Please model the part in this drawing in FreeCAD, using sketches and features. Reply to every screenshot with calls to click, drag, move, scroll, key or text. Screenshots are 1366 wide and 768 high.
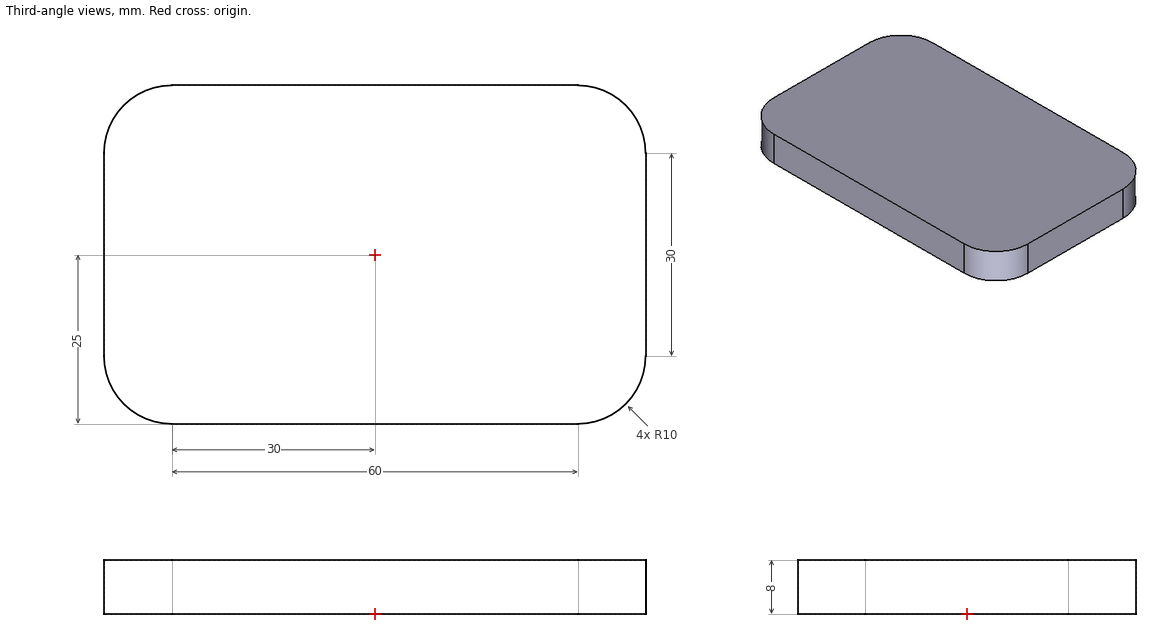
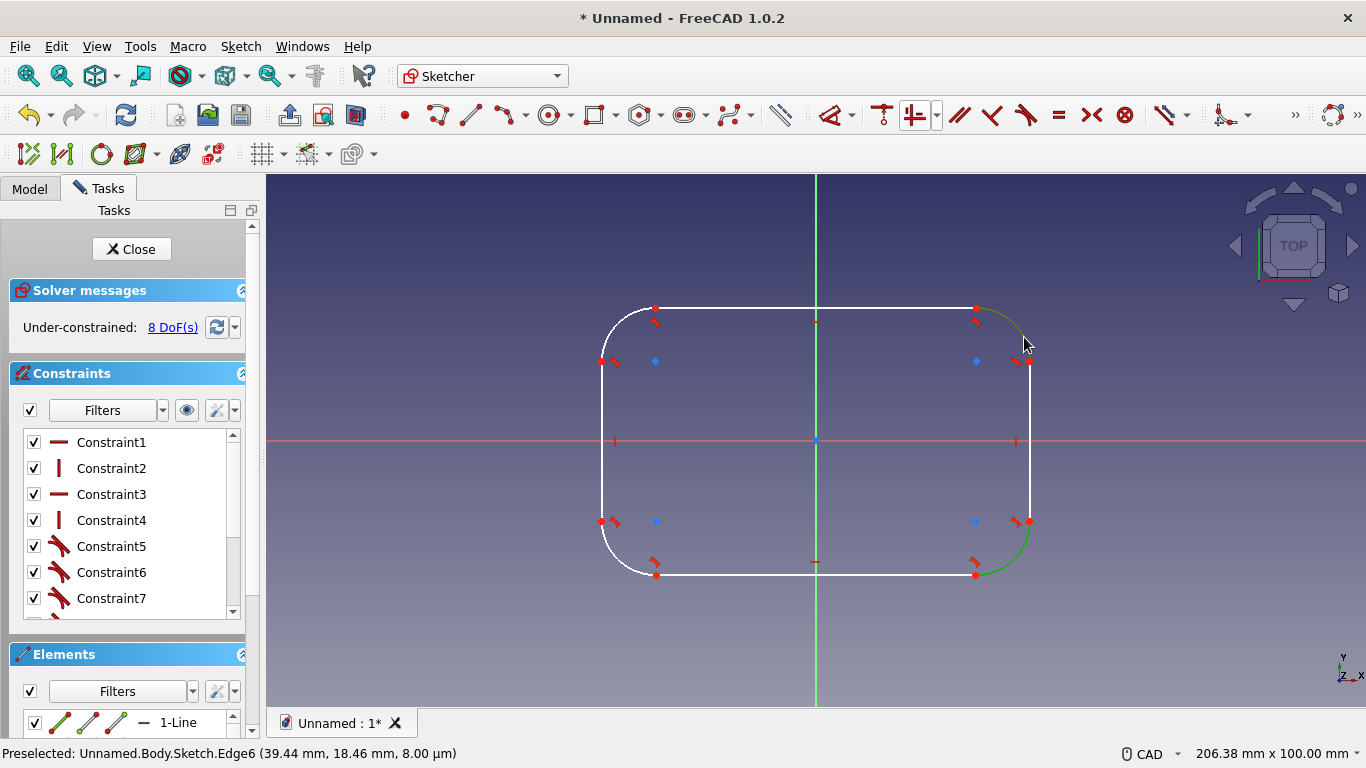
click(631, 314)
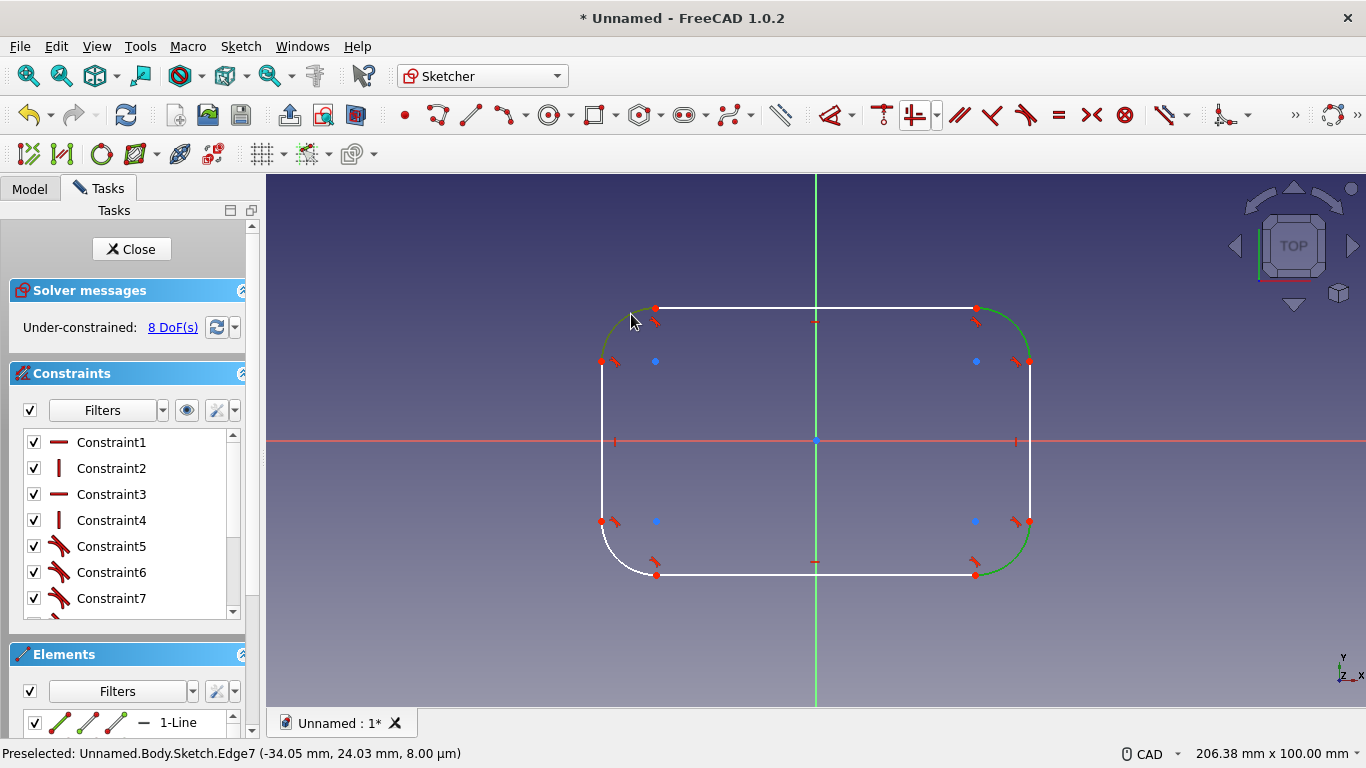
click(608, 546)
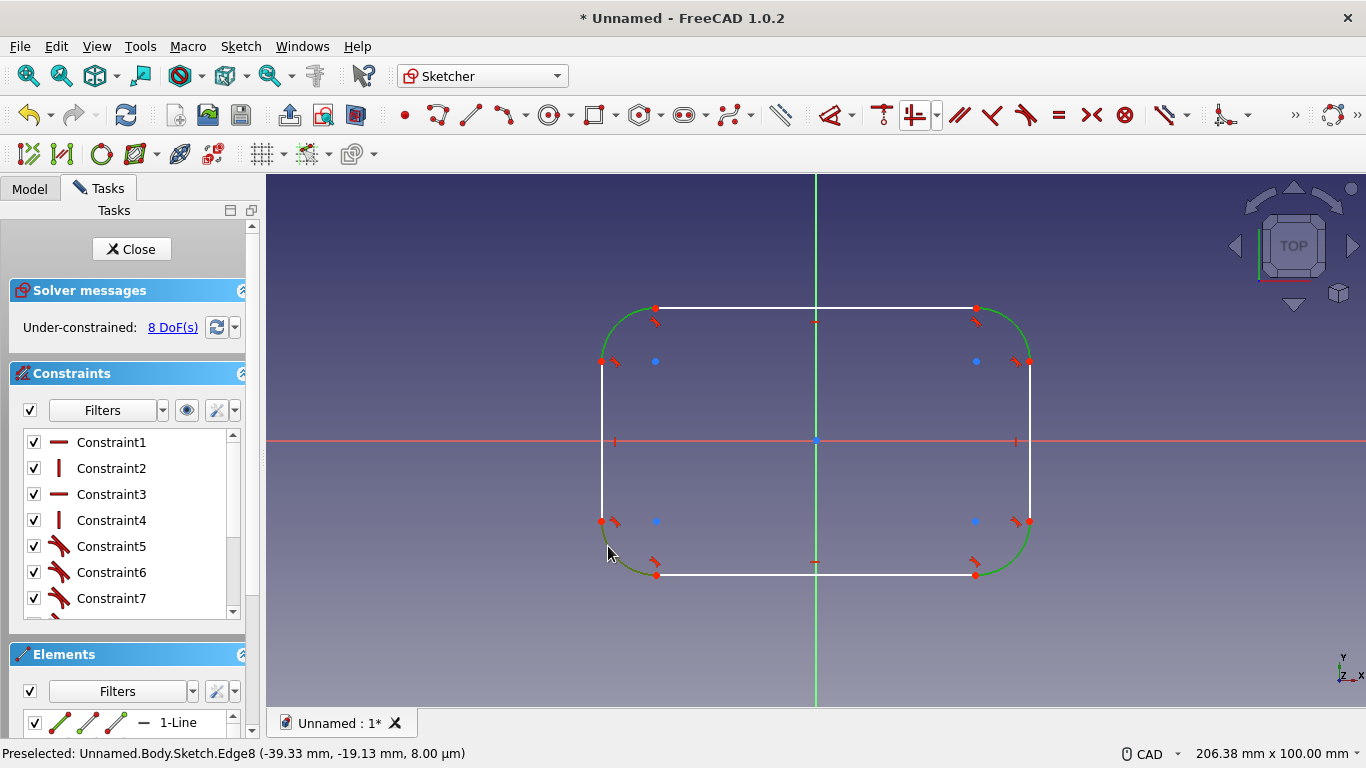
key(e)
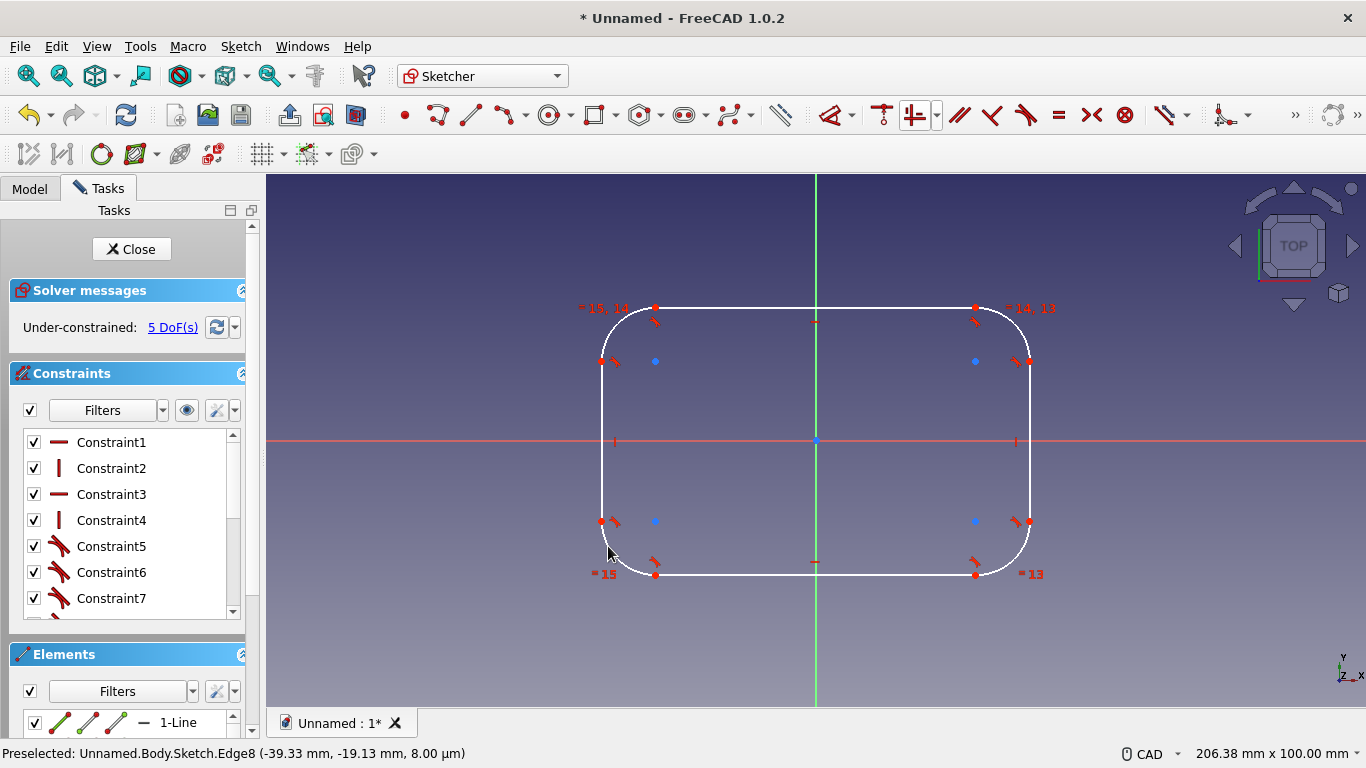
click(830, 116)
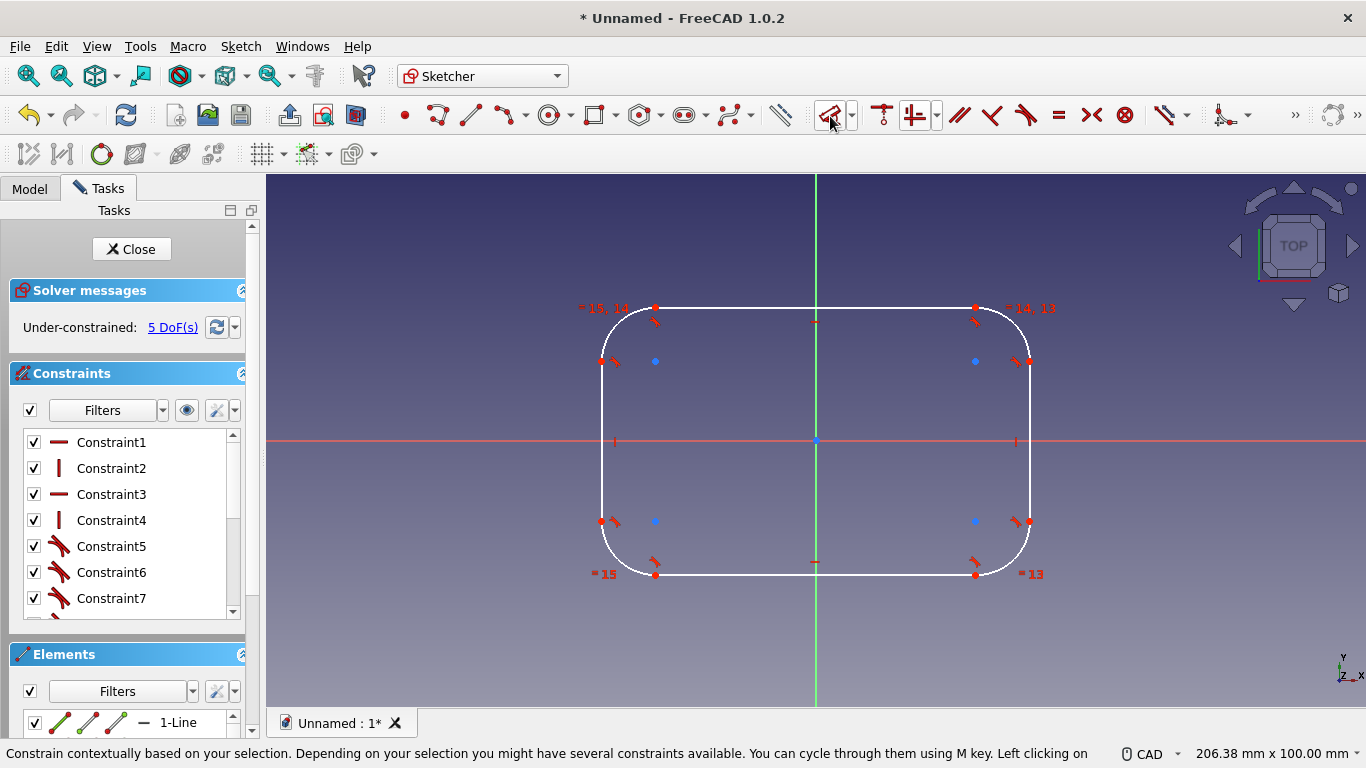
click(1000, 569)
click(1014, 598)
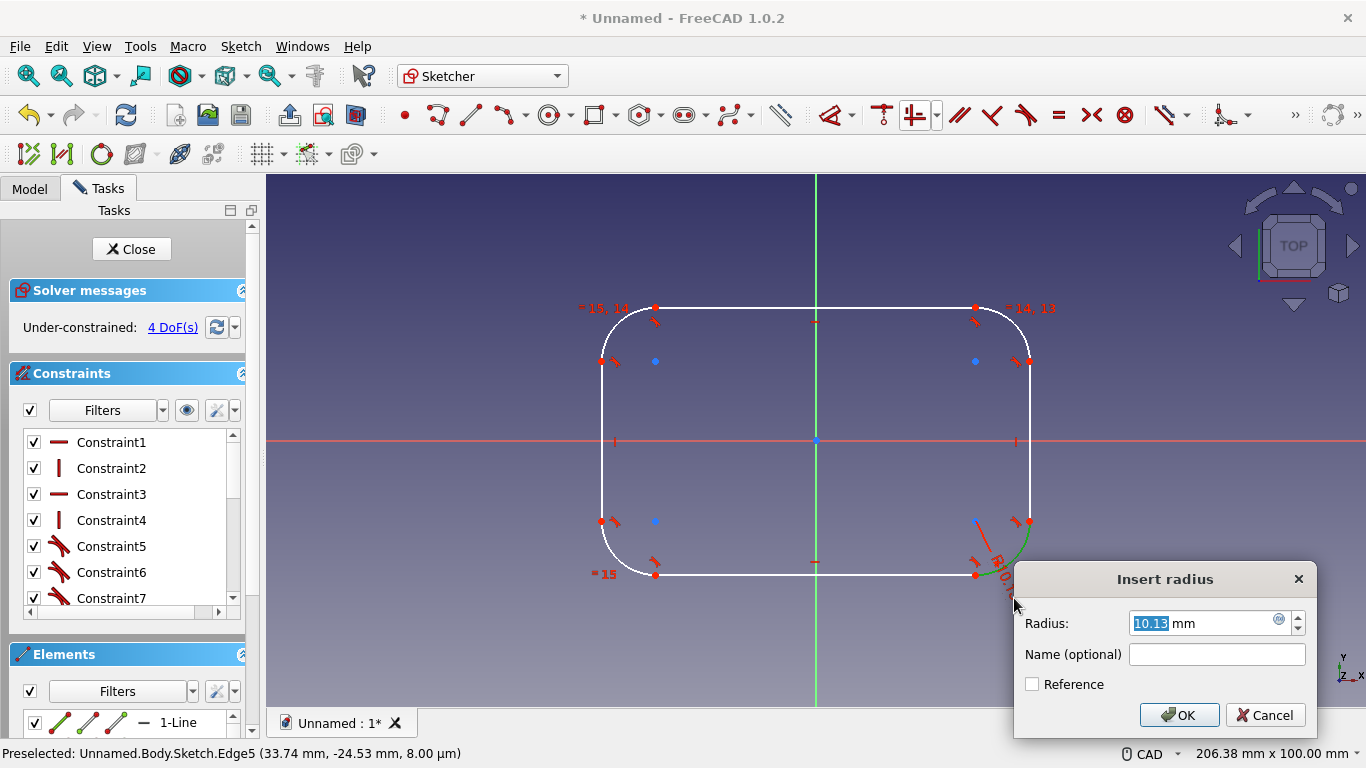
text(10)
key(Return)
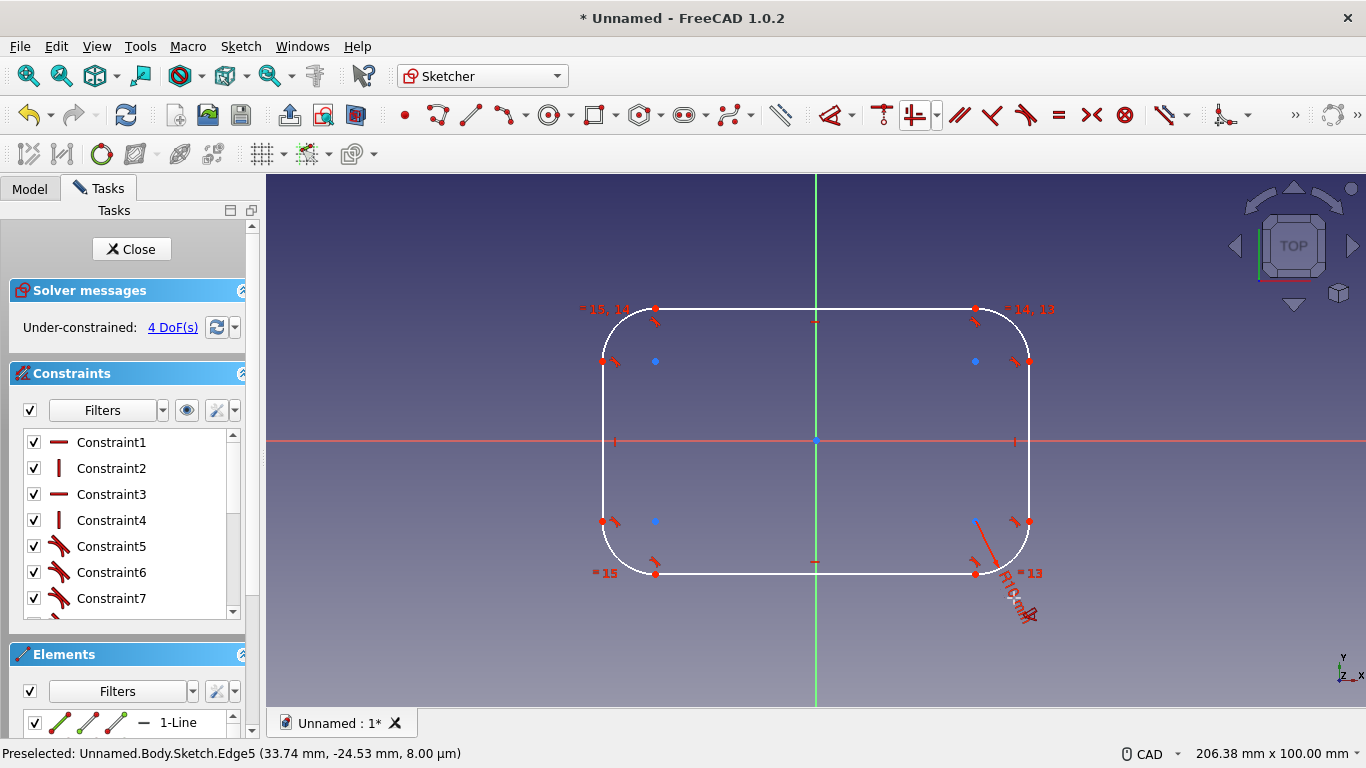
click(752, 574)
click(742, 608)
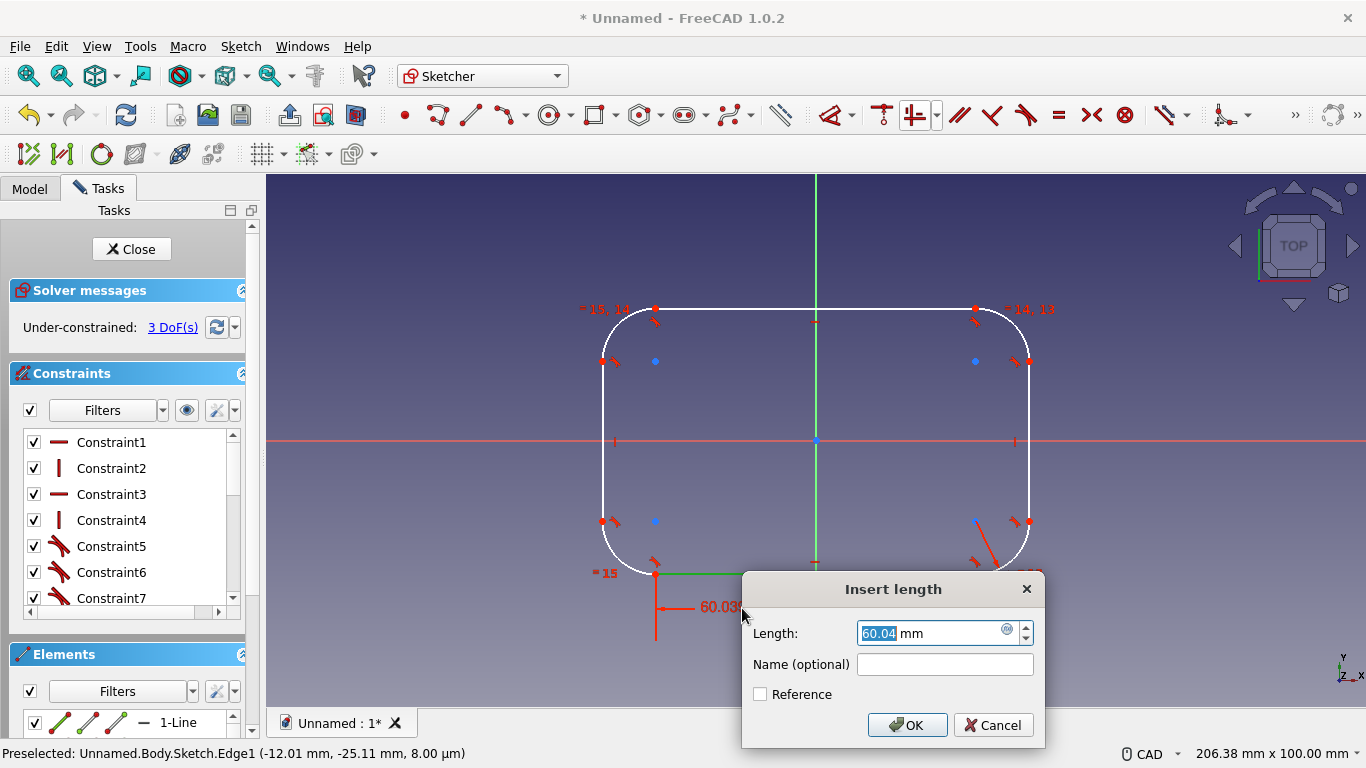
text(60)
key(Return)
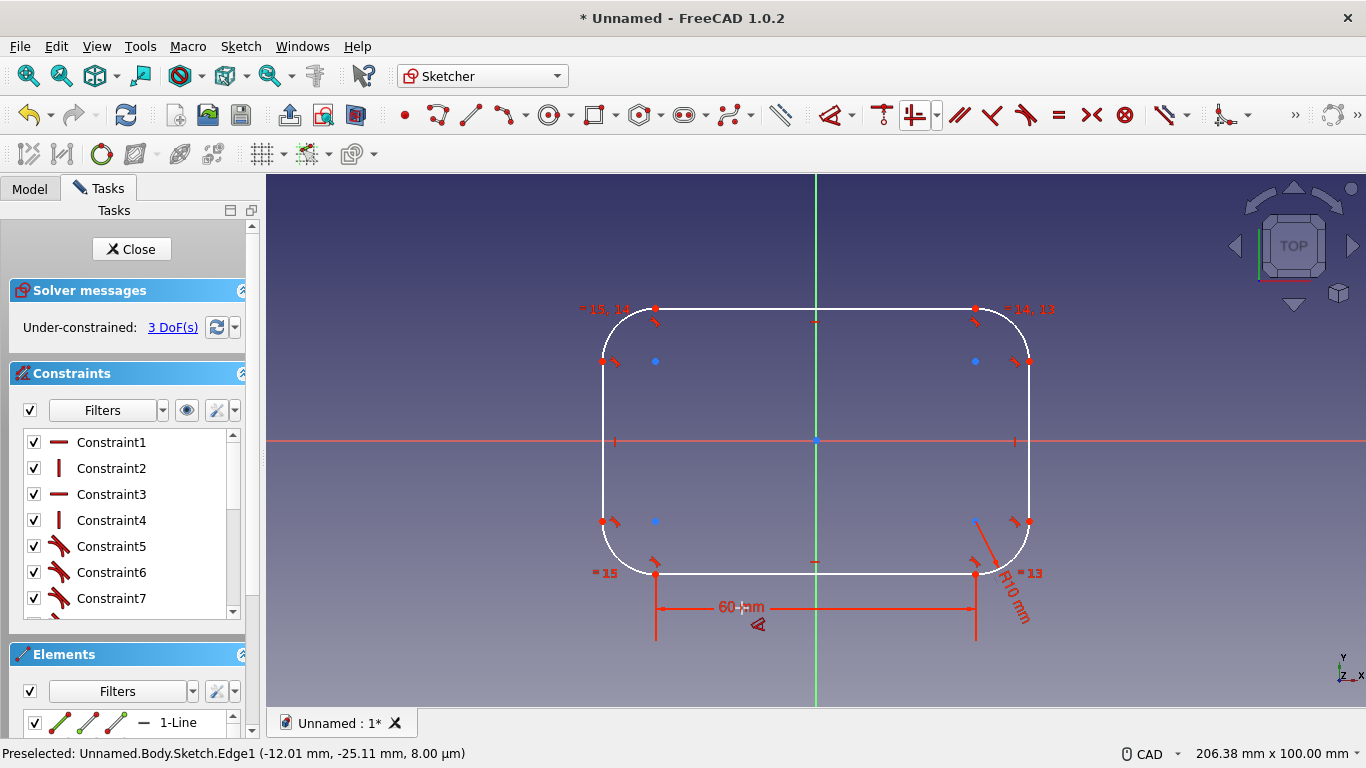
click(1029, 473)
click(1063, 405)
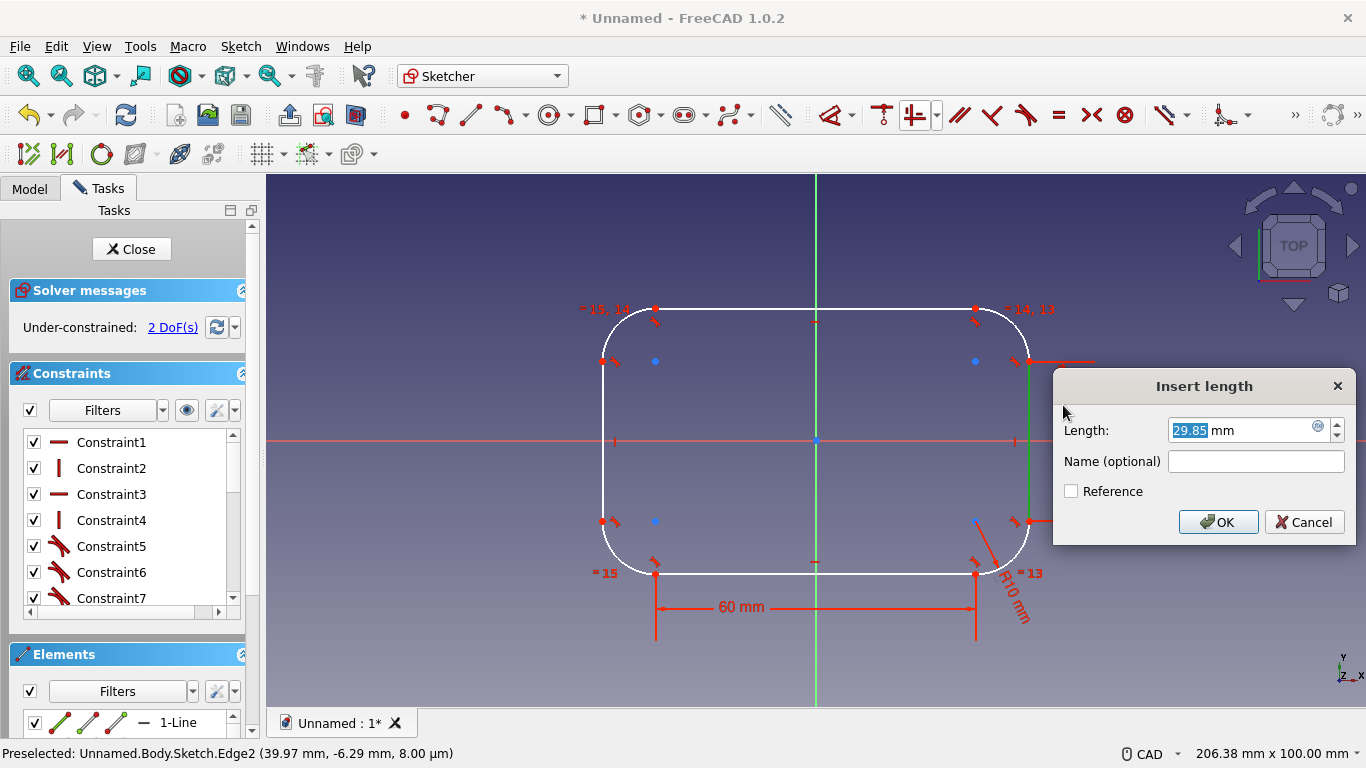
text(30)
key(Return)